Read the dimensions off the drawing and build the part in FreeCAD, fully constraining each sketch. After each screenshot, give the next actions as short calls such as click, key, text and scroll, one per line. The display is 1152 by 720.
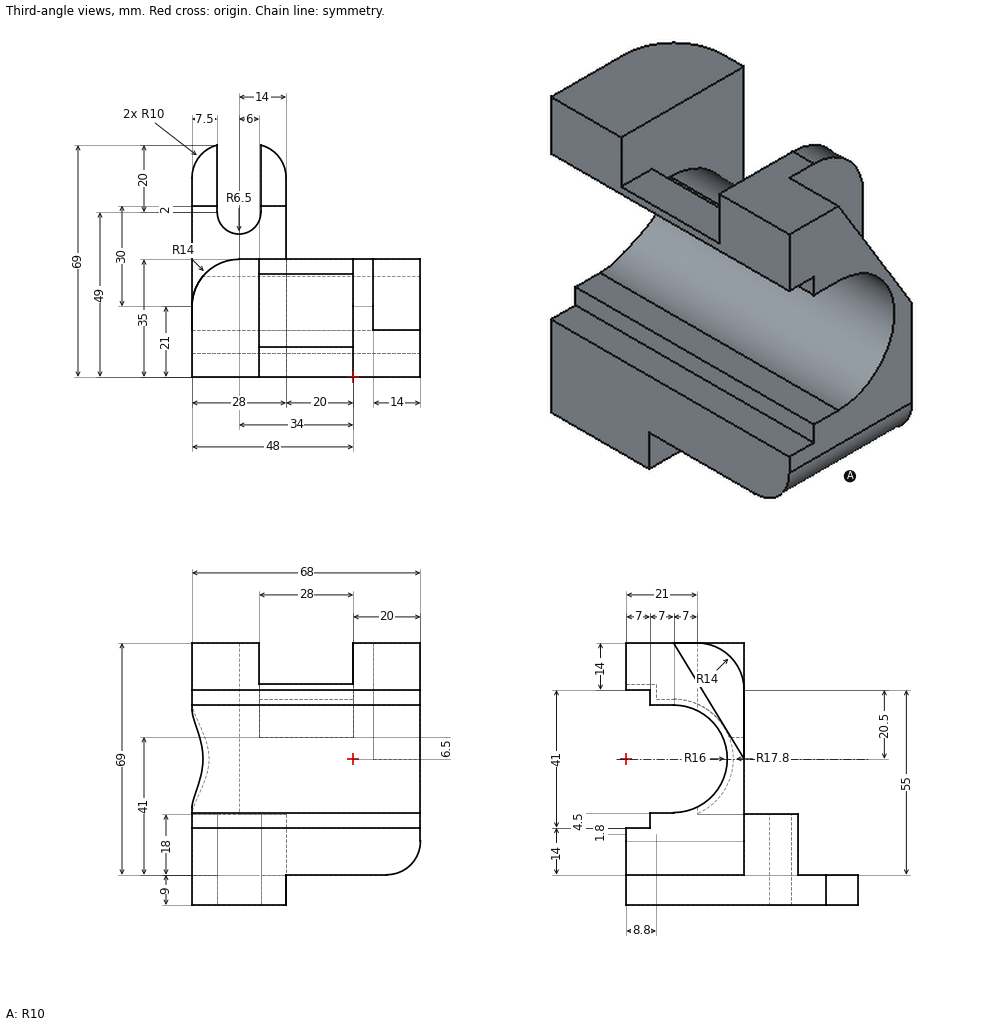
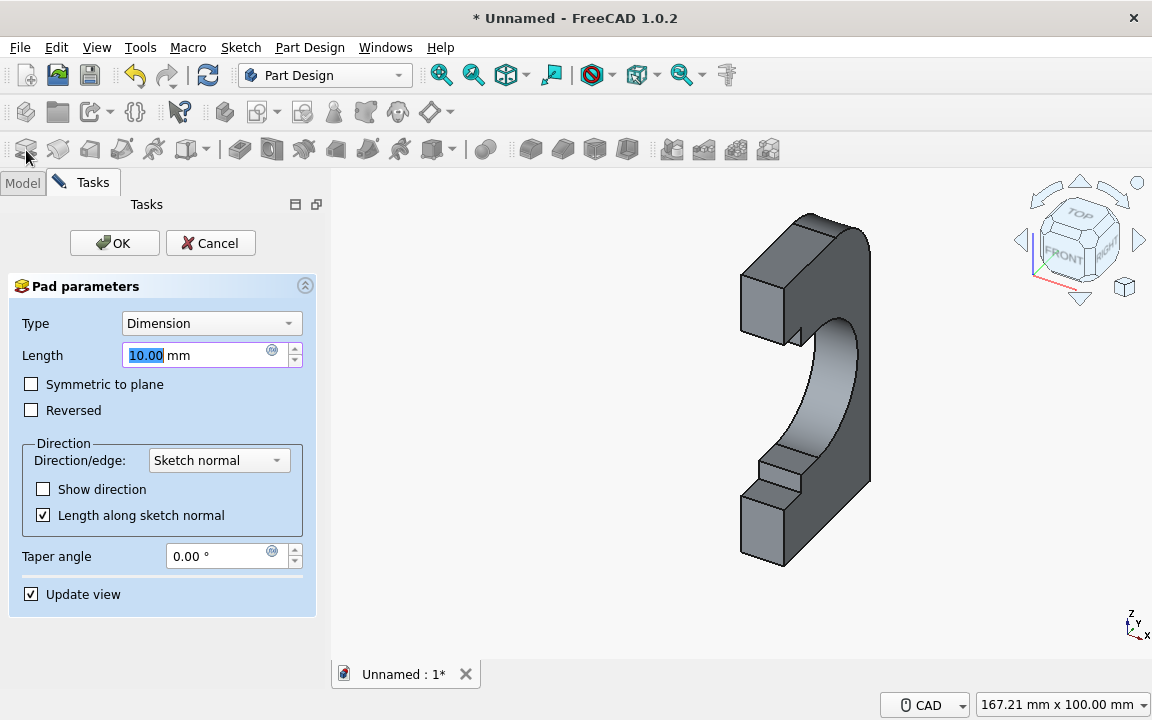
text(20)
key(Tab)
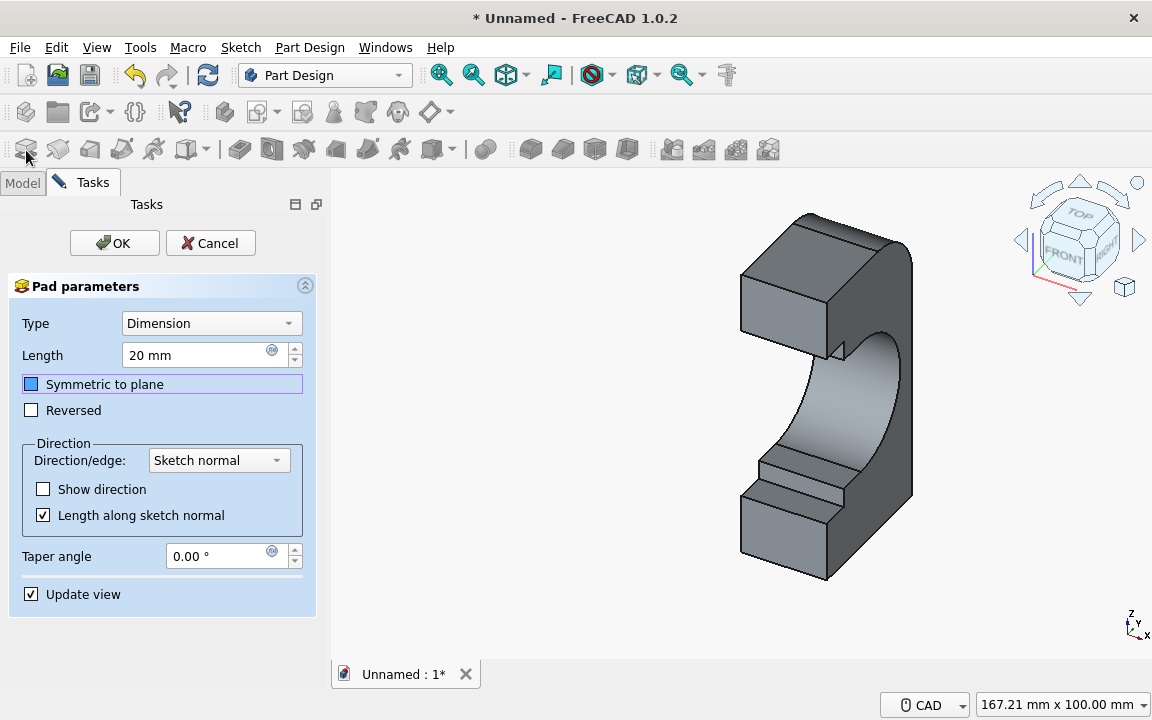
click(115, 243)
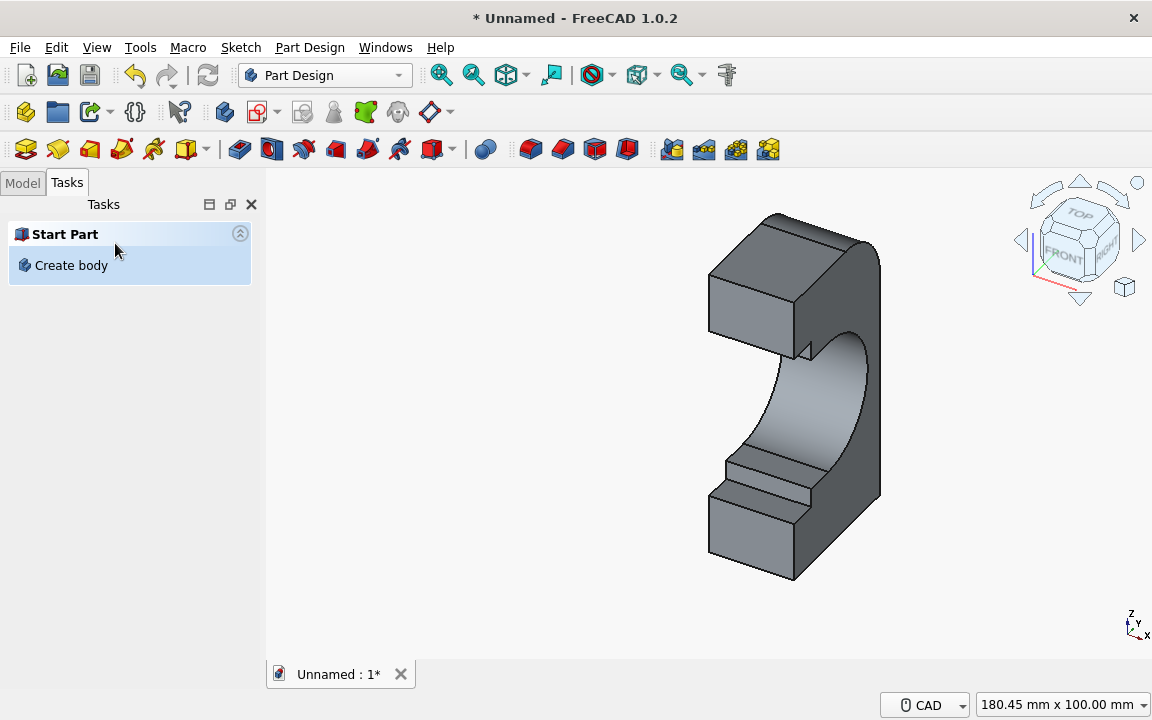
click(23, 182)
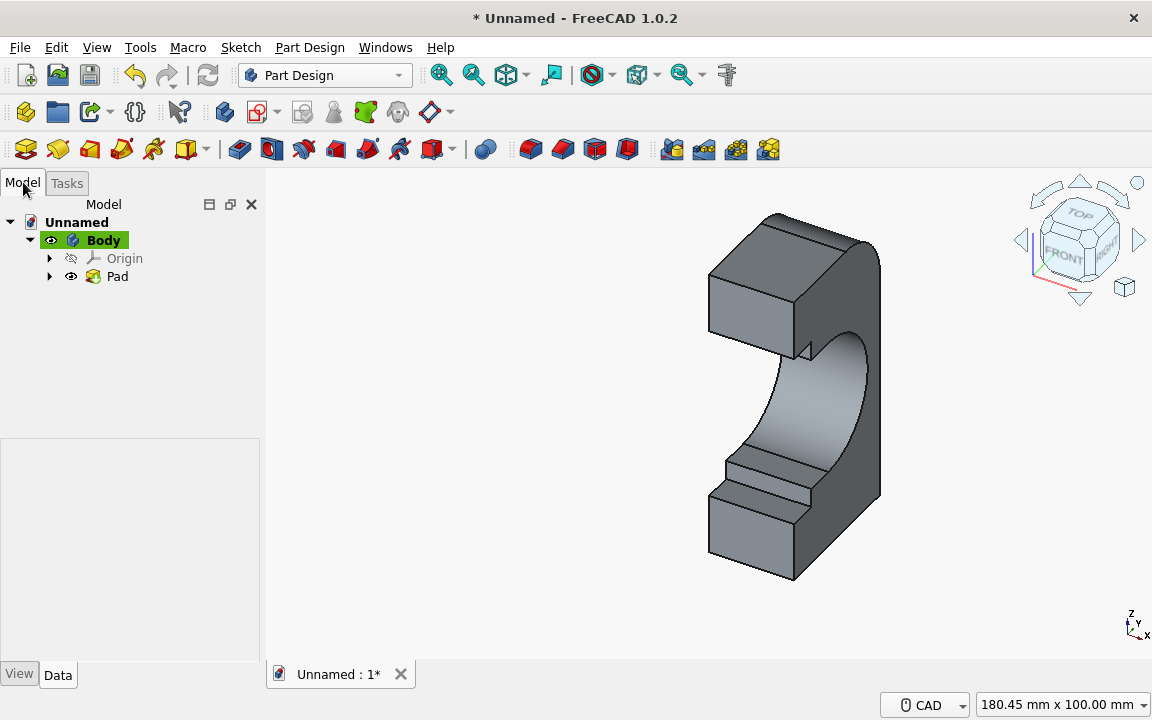
click(50, 258)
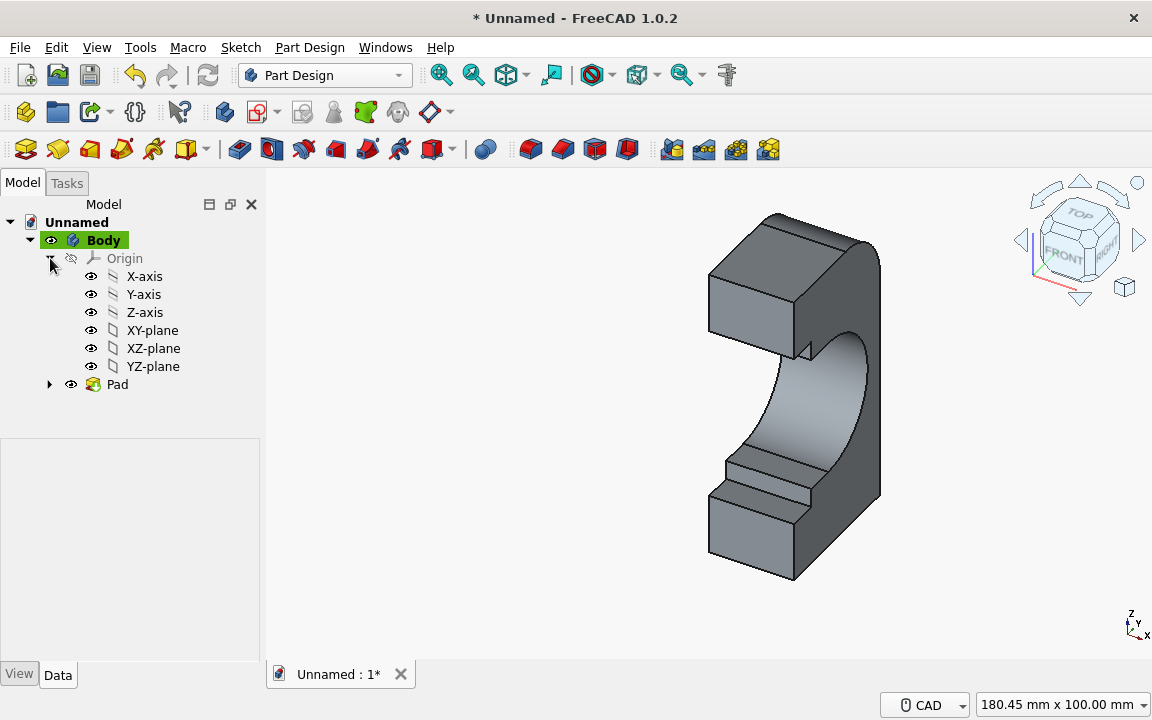
click(136, 366)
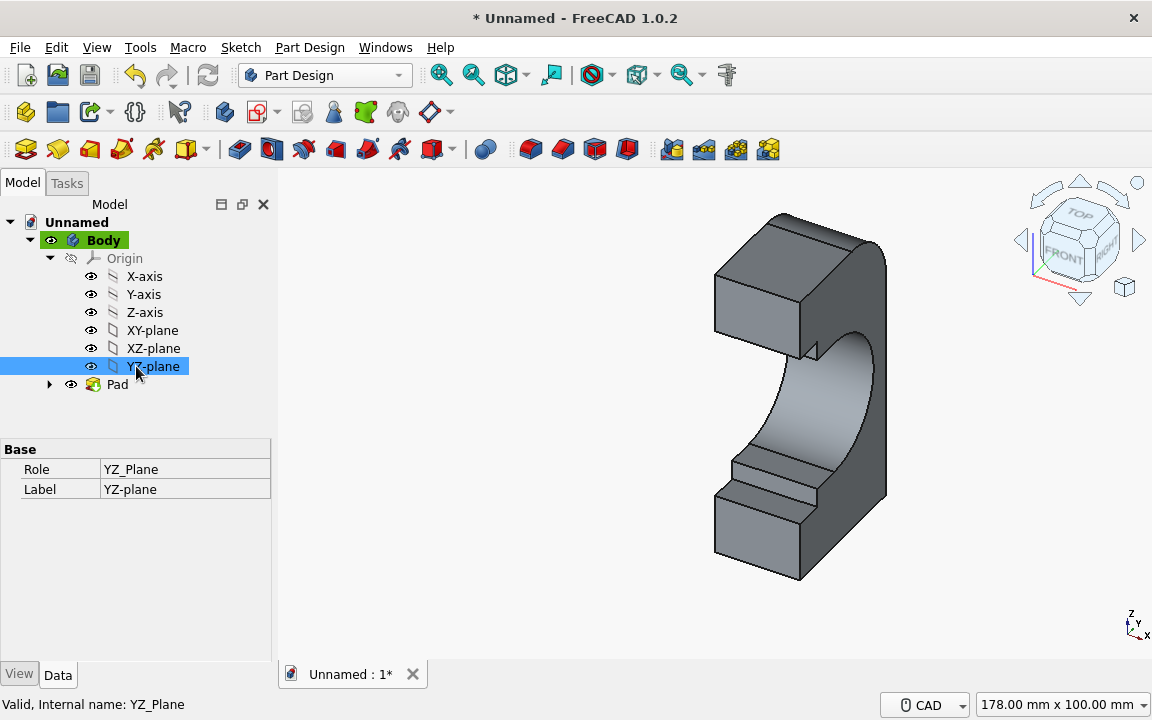
click(430, 112)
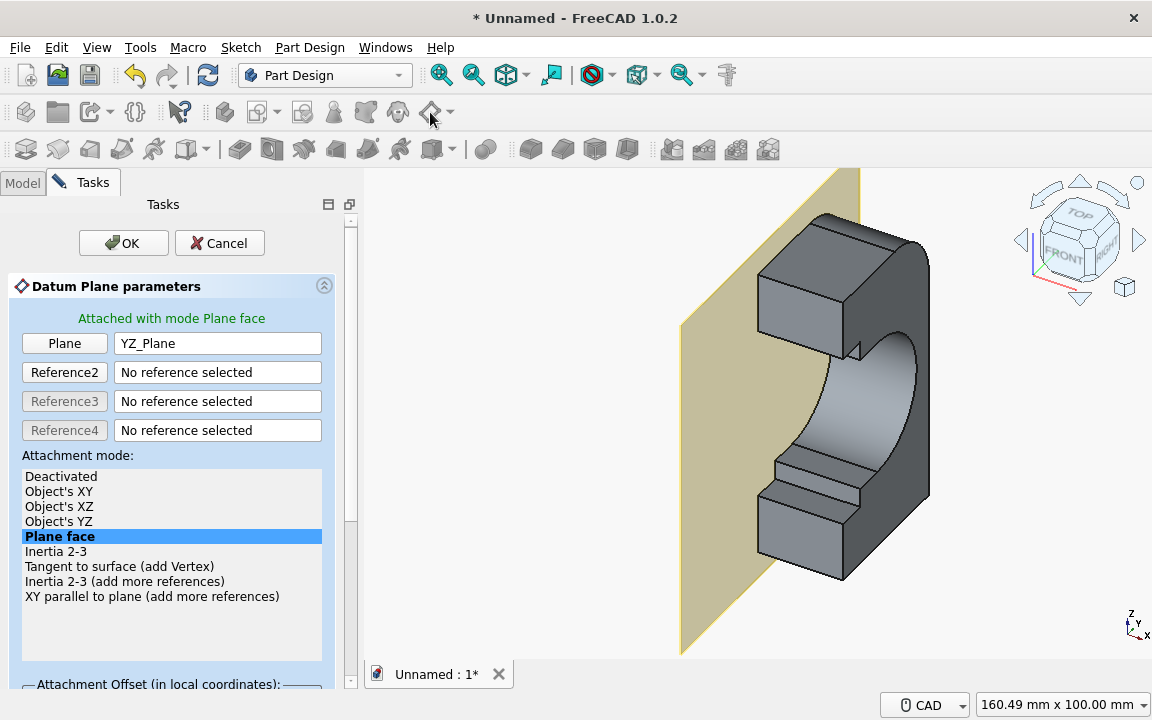
scroll(351, 451, down, 3)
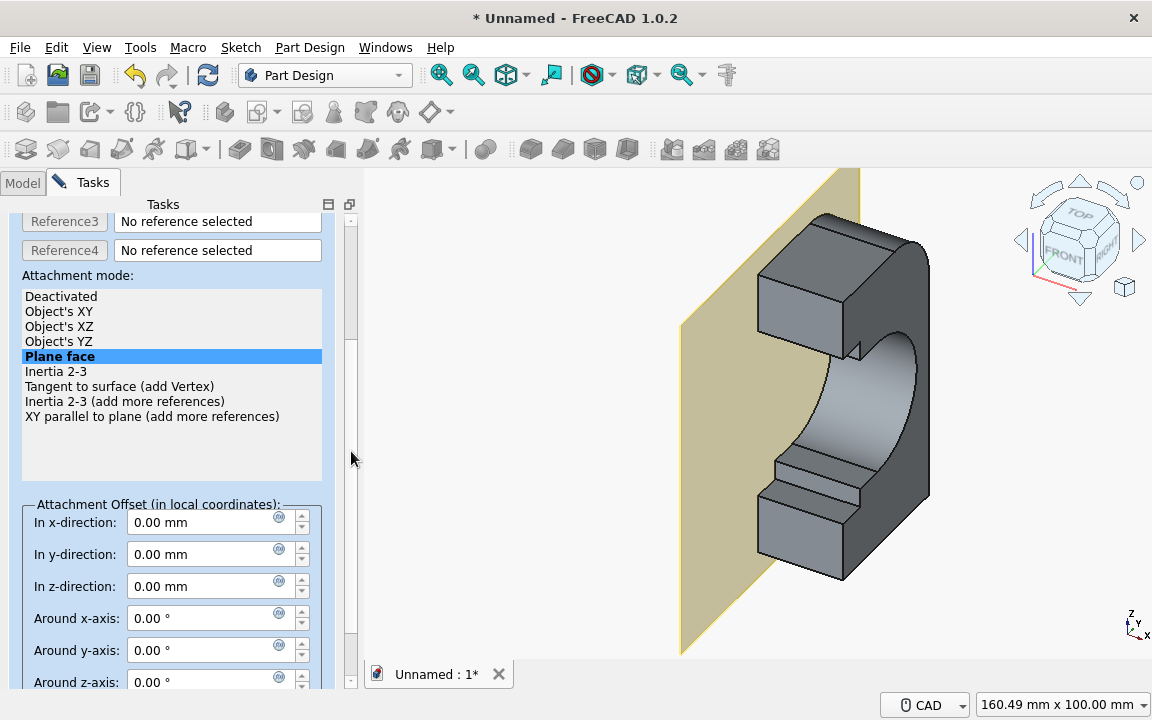
triple_click(210, 586)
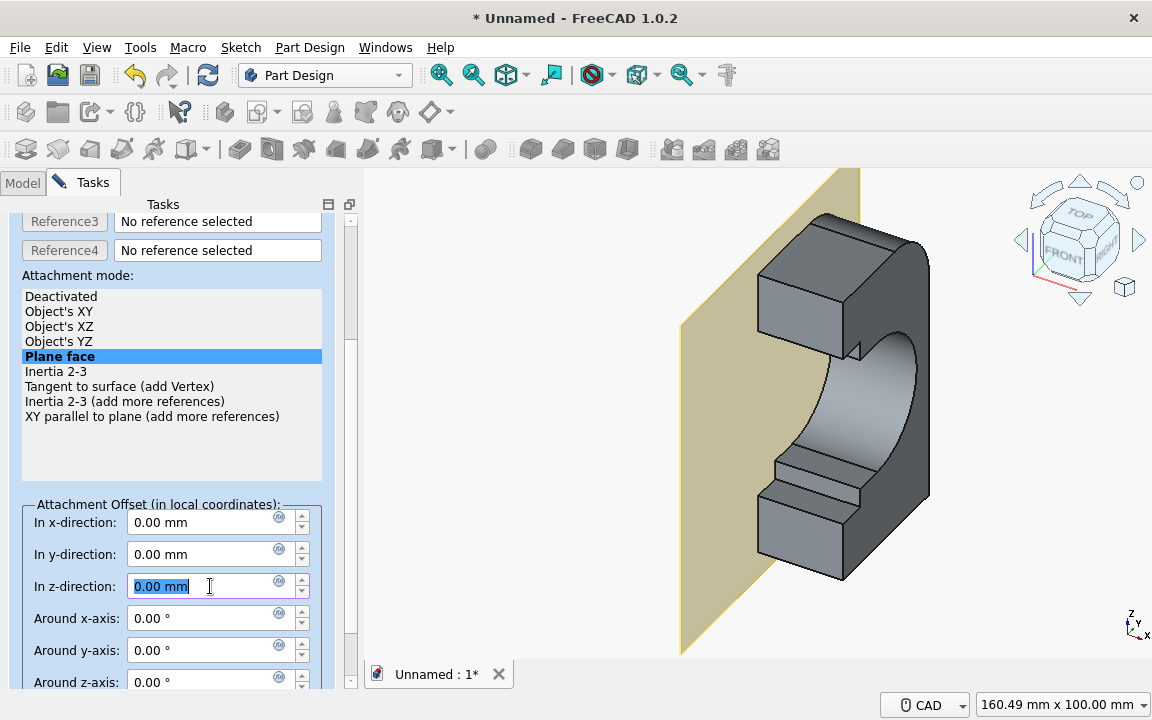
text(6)
key(Tab)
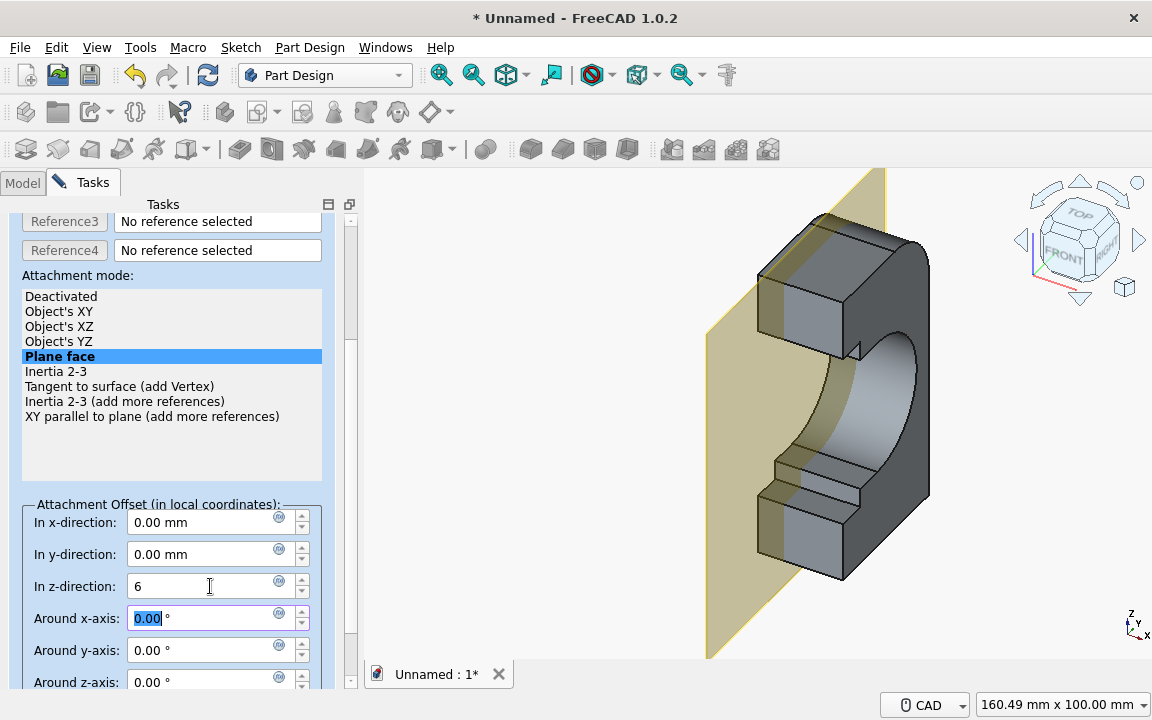
scroll(351, 451, up, 4)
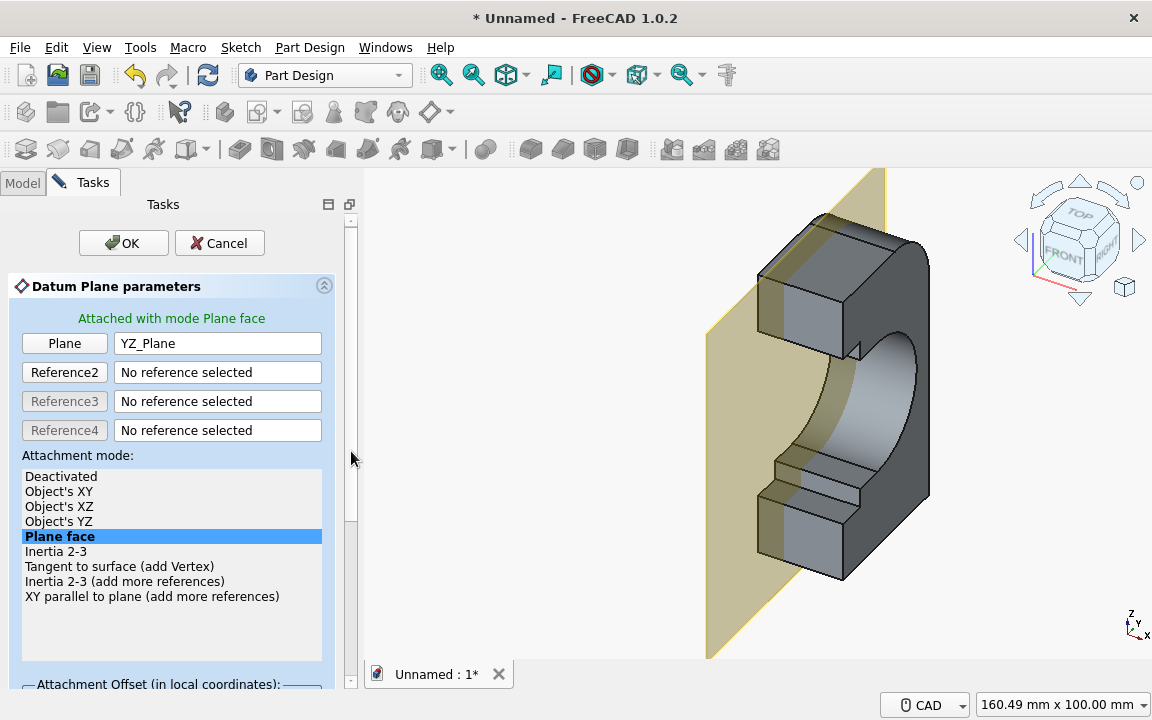
click(124, 243)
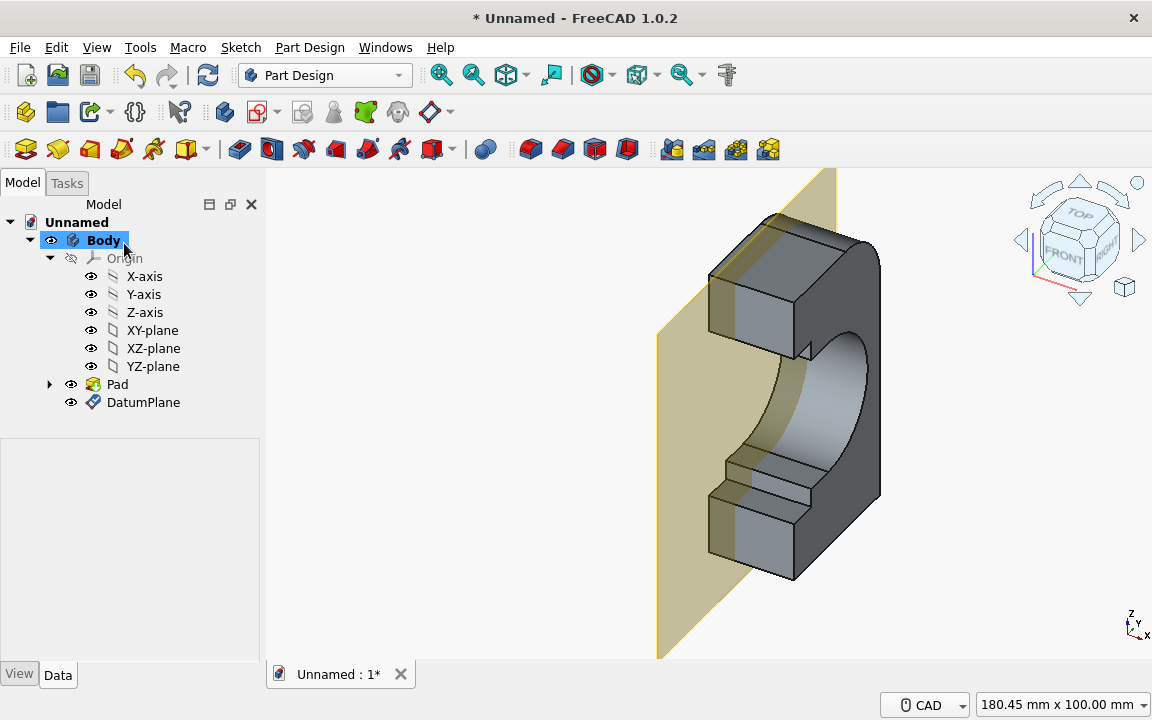
click(116, 402)